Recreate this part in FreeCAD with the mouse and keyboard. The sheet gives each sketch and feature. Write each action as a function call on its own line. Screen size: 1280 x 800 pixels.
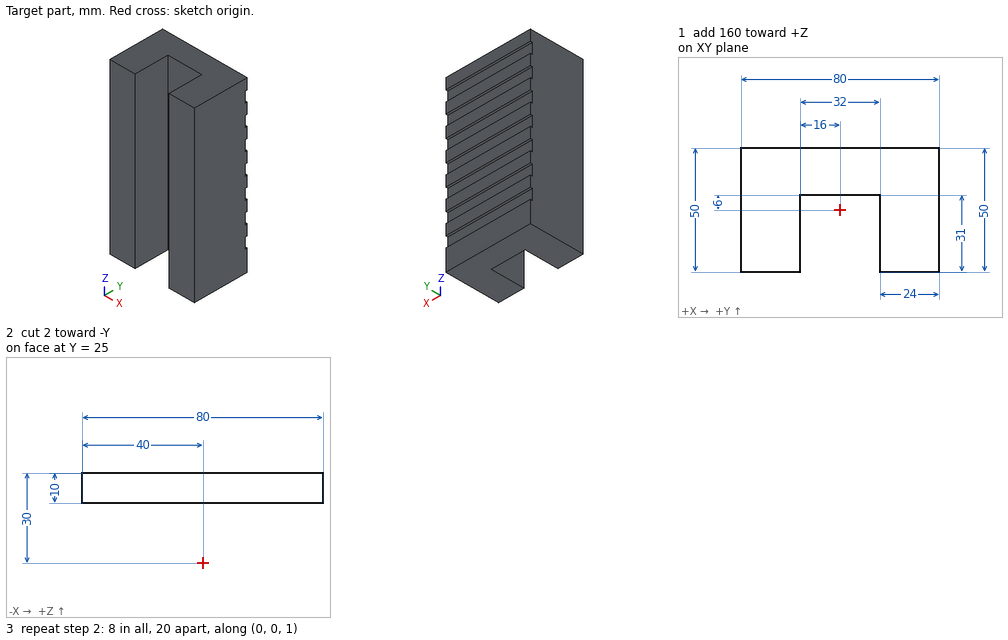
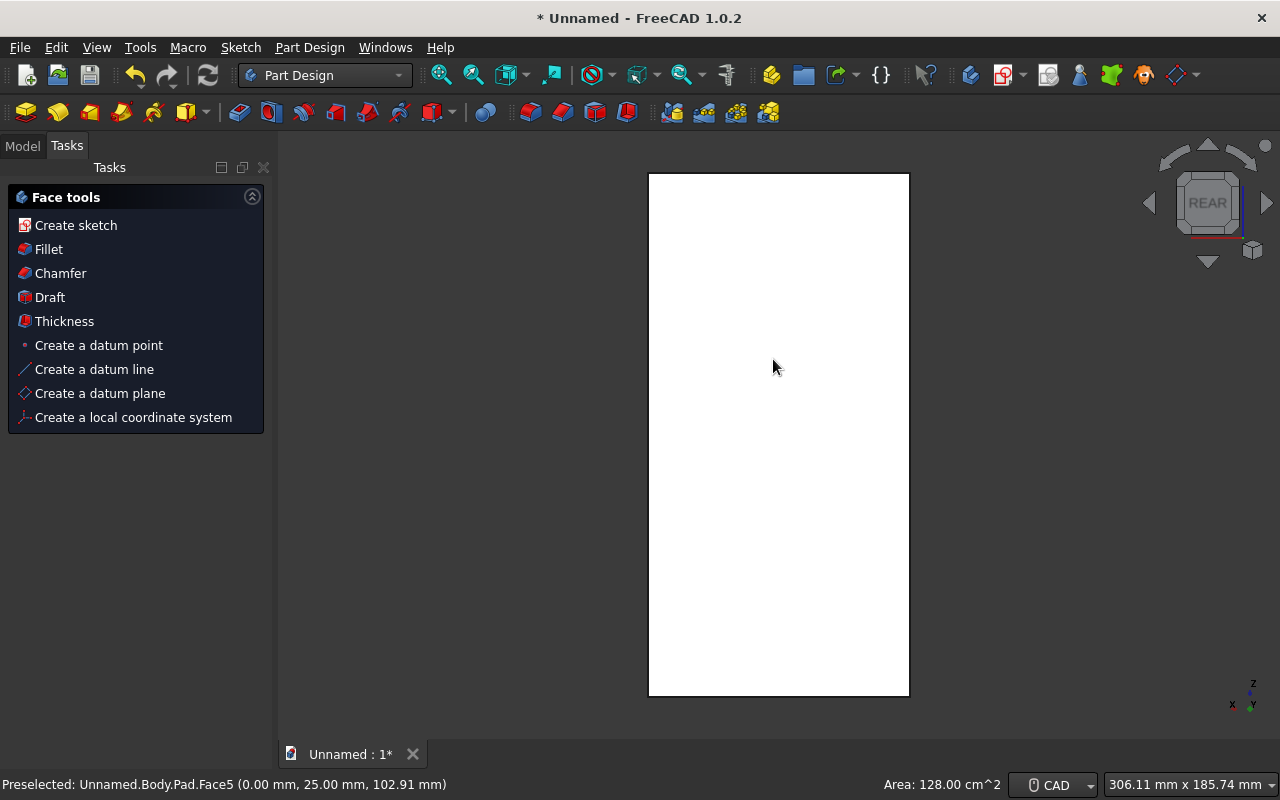
click(1004, 76)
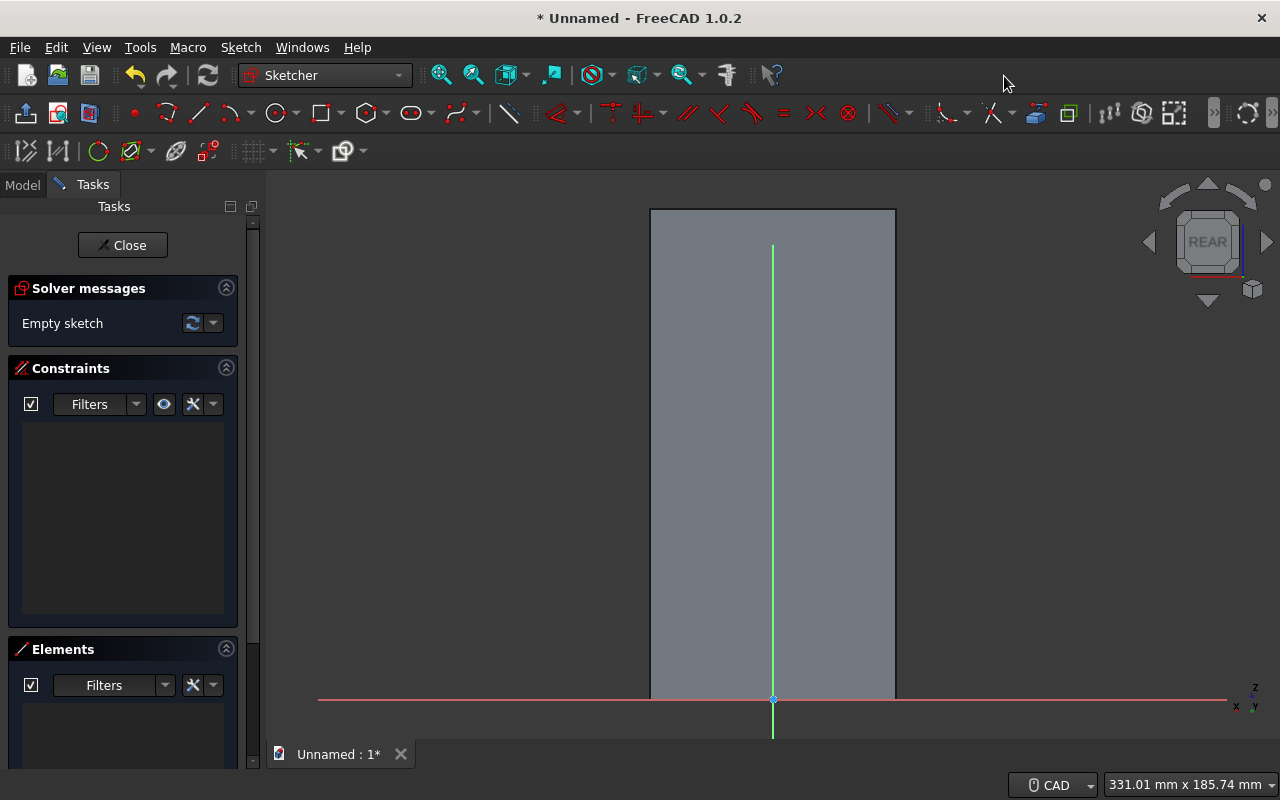
scroll(829, 711, up, 4)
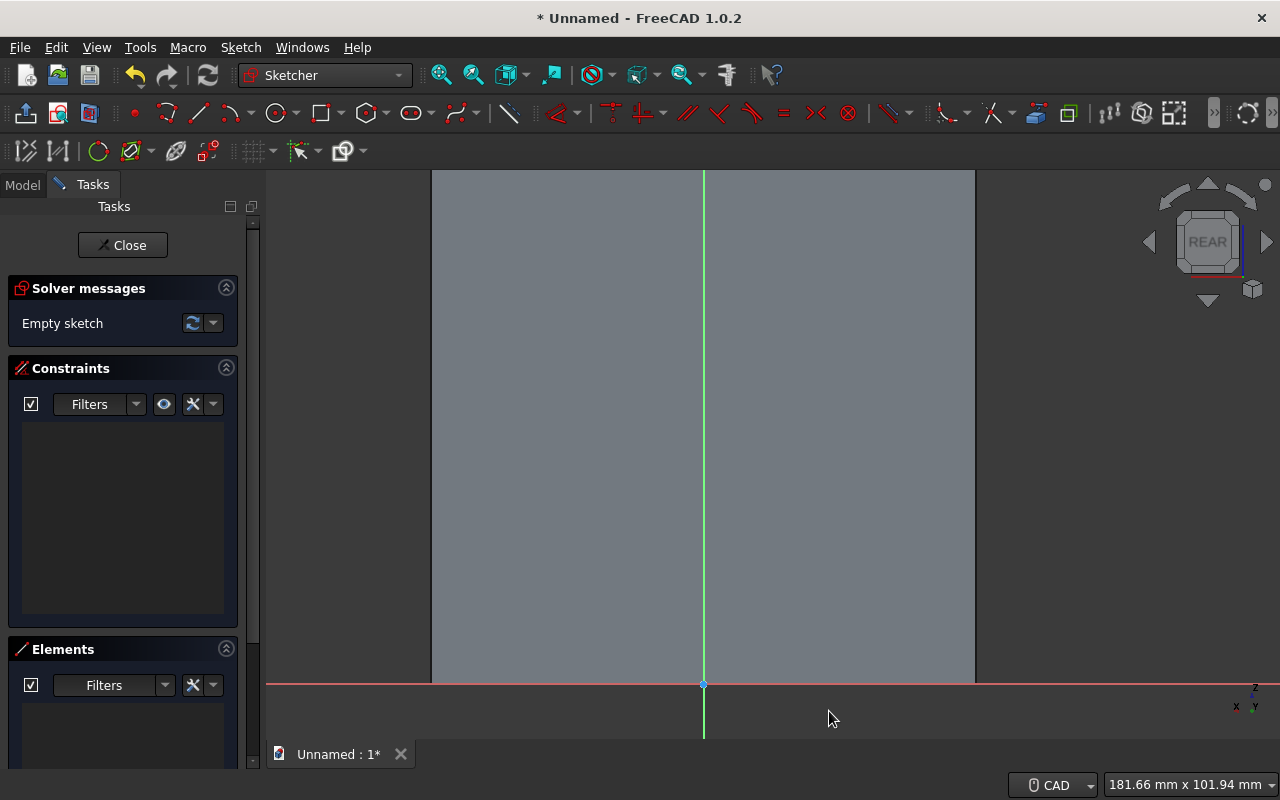
click(322, 114)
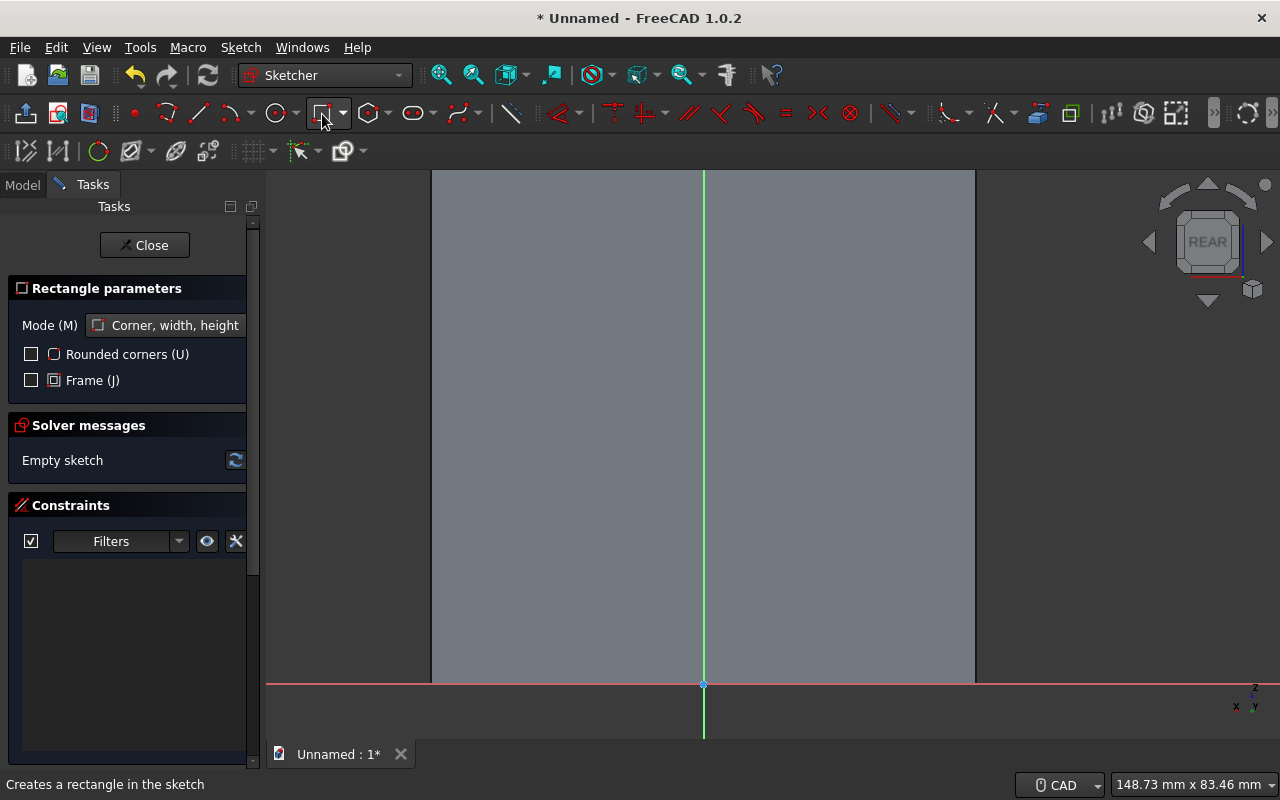
click(431, 480)
click(976, 548)
key(Escape)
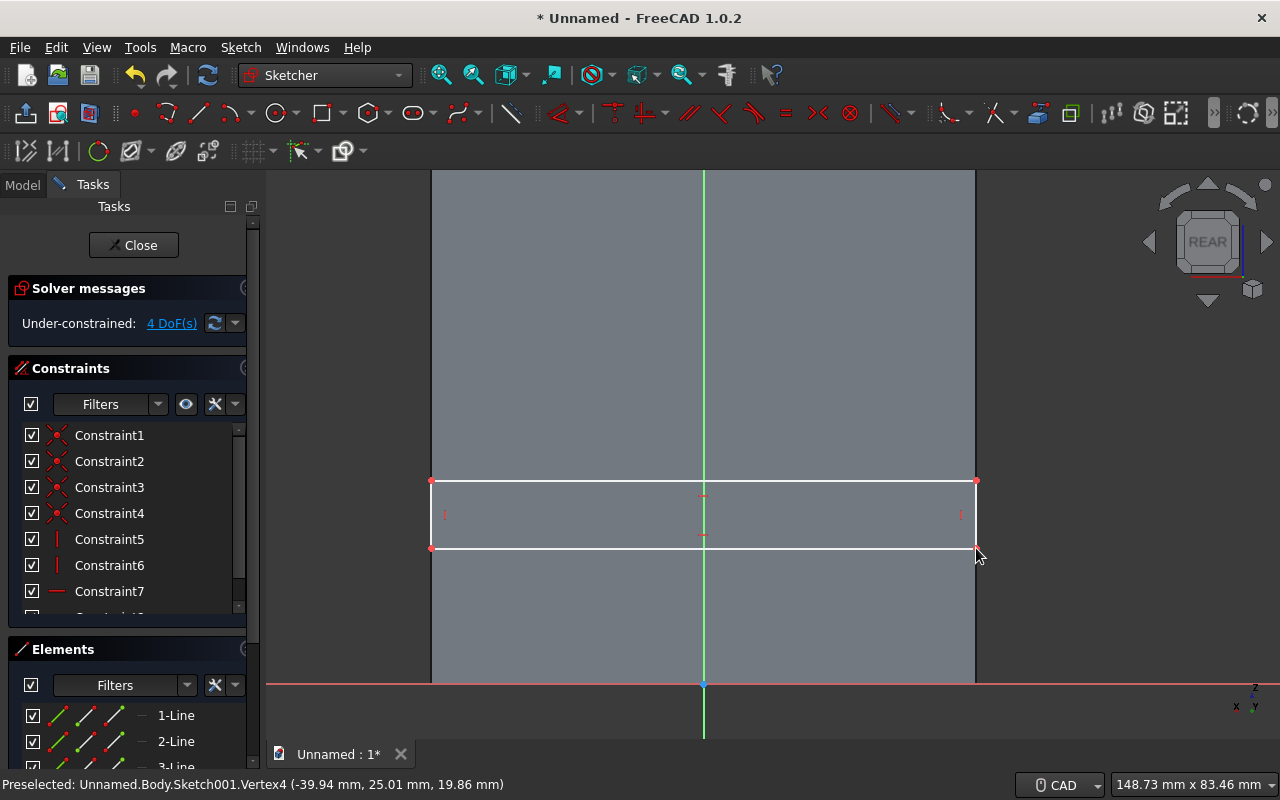
click(558, 114)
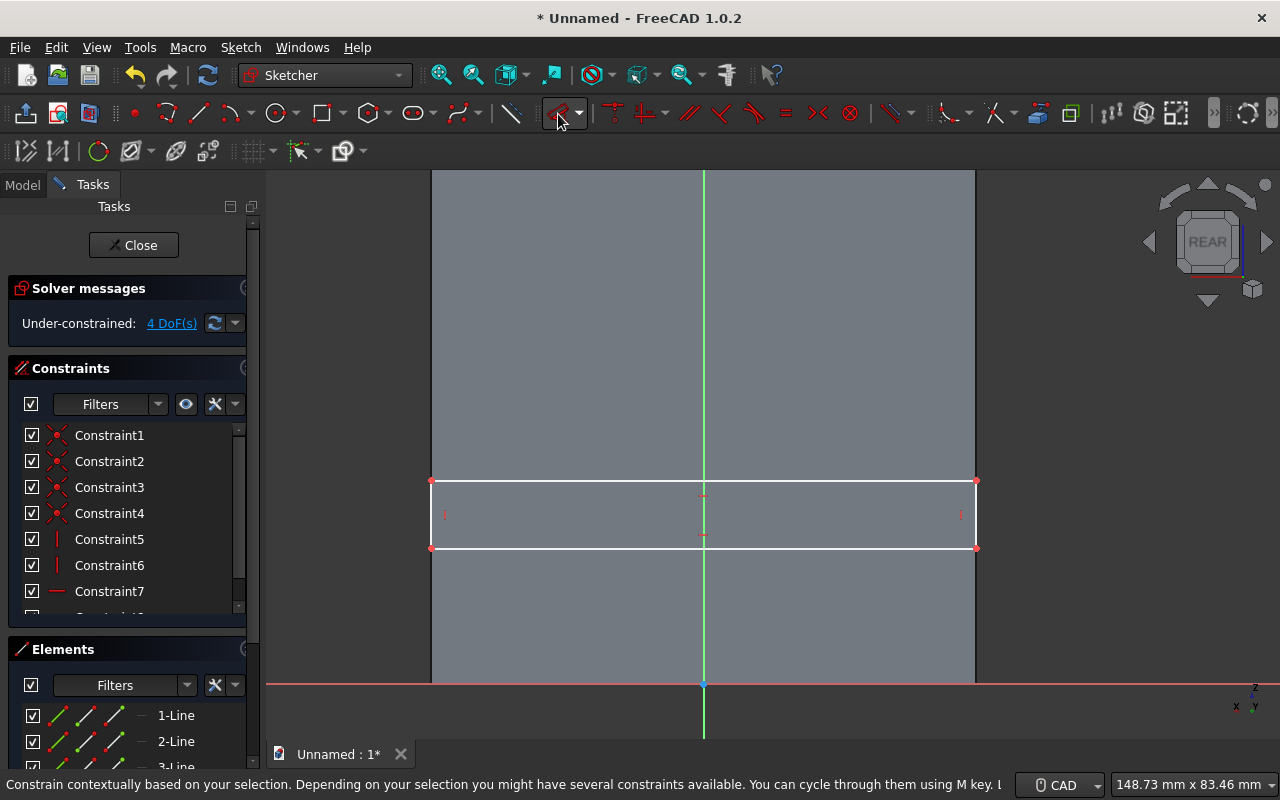
click(431, 501)
click(397, 515)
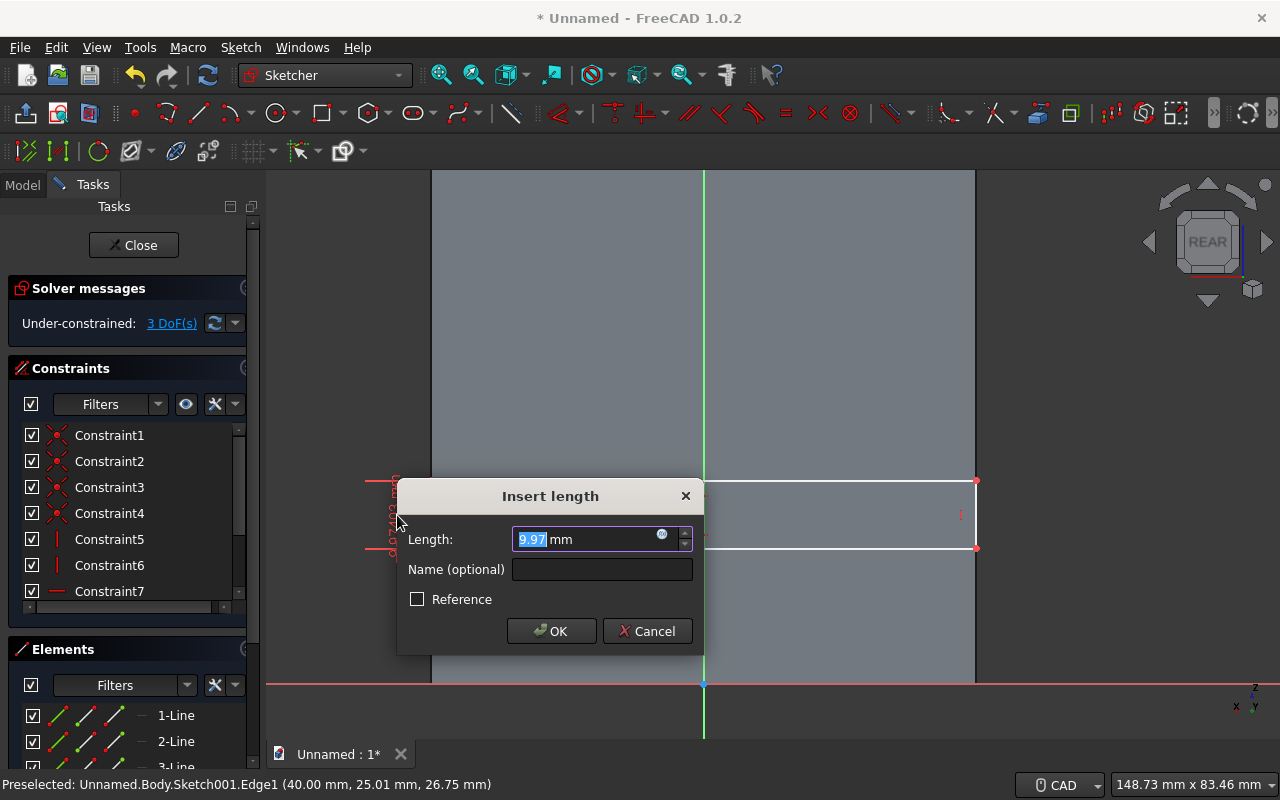
text(10)
key(Return)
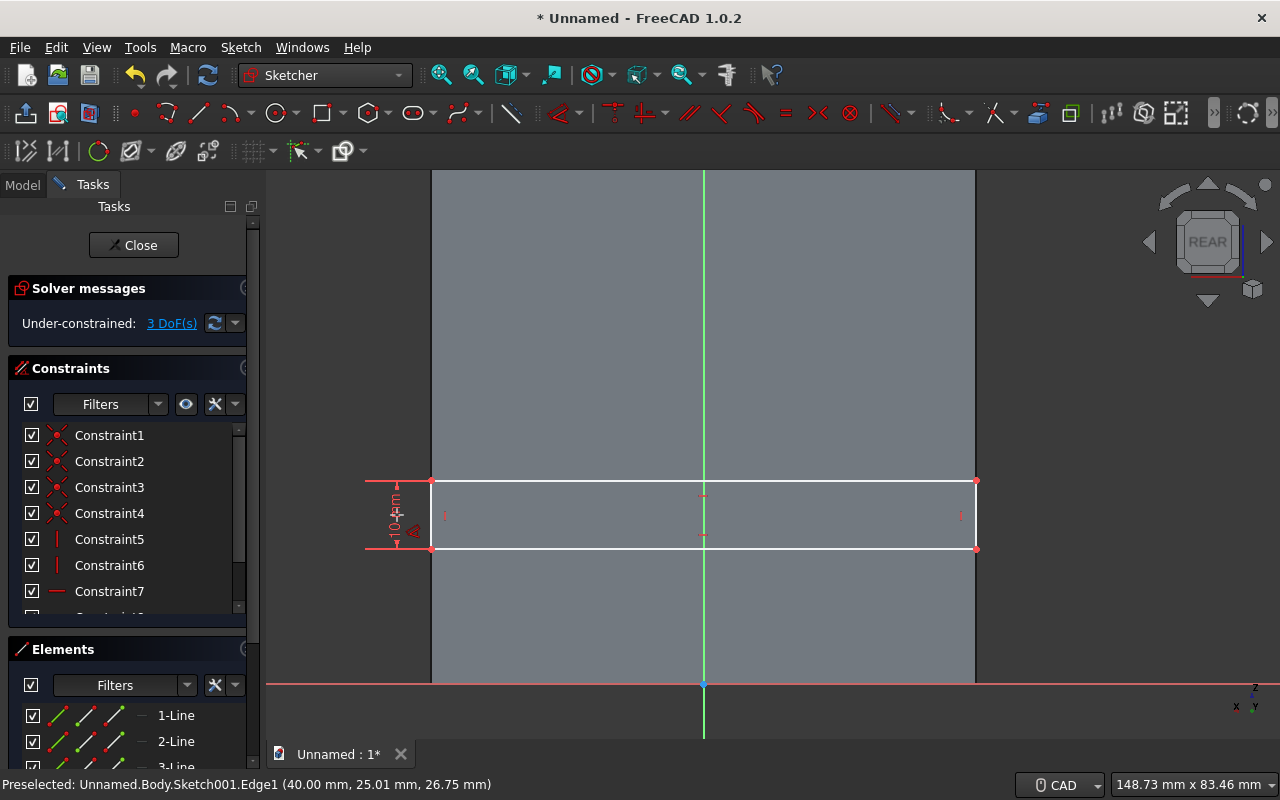
click(594, 549)
click(578, 515)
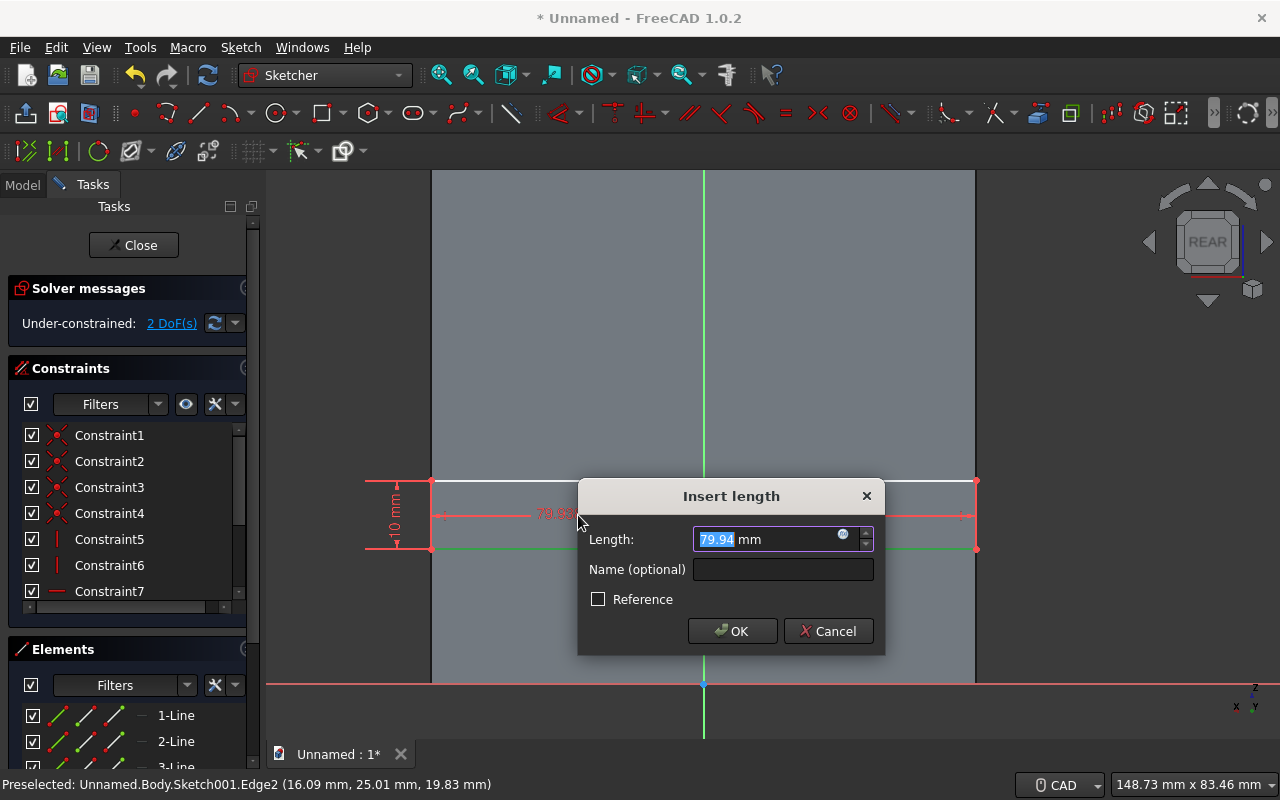
text(80)
key(Return)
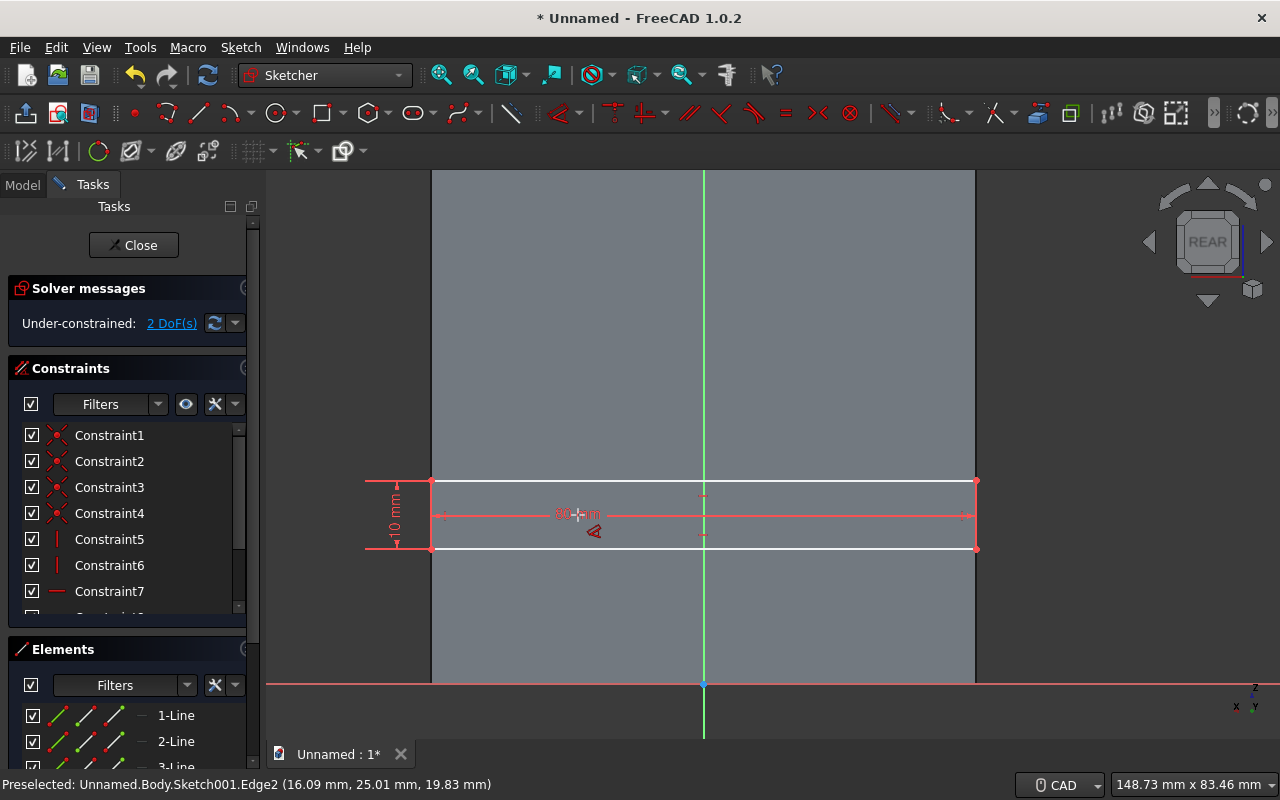
click(431, 481)
click(567, 447)